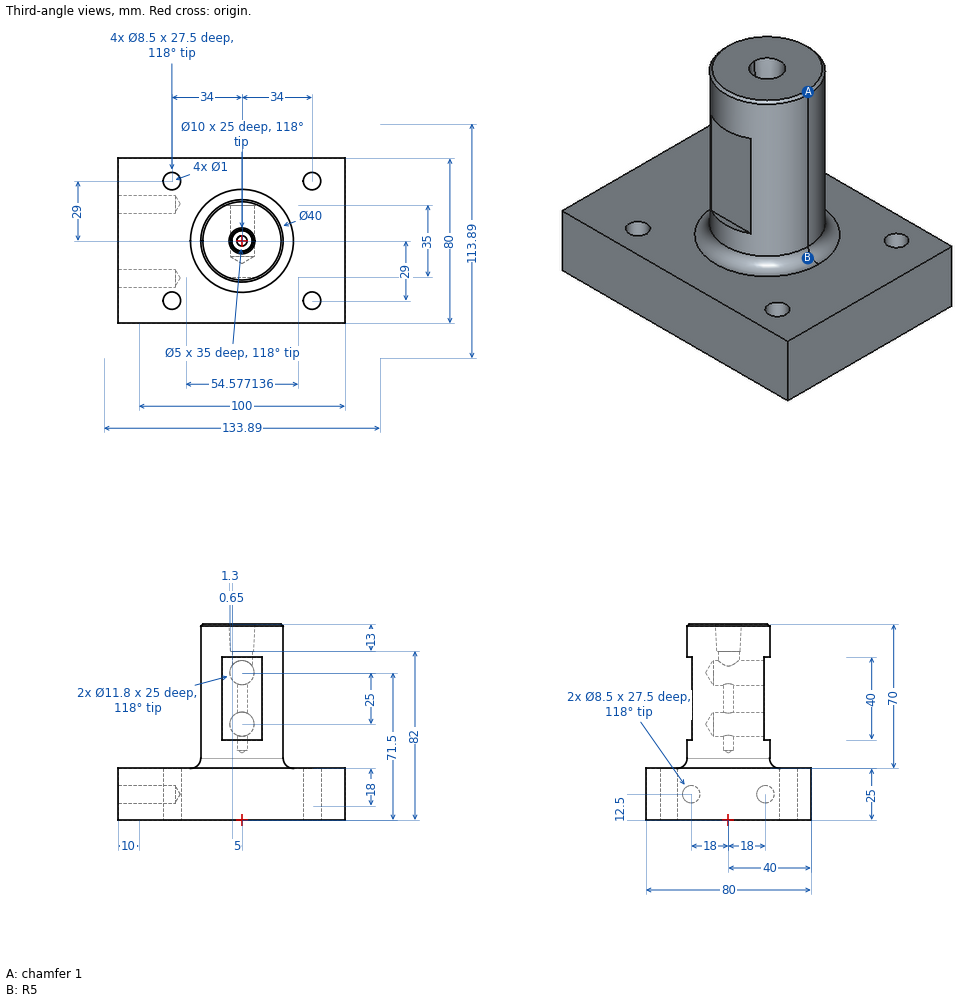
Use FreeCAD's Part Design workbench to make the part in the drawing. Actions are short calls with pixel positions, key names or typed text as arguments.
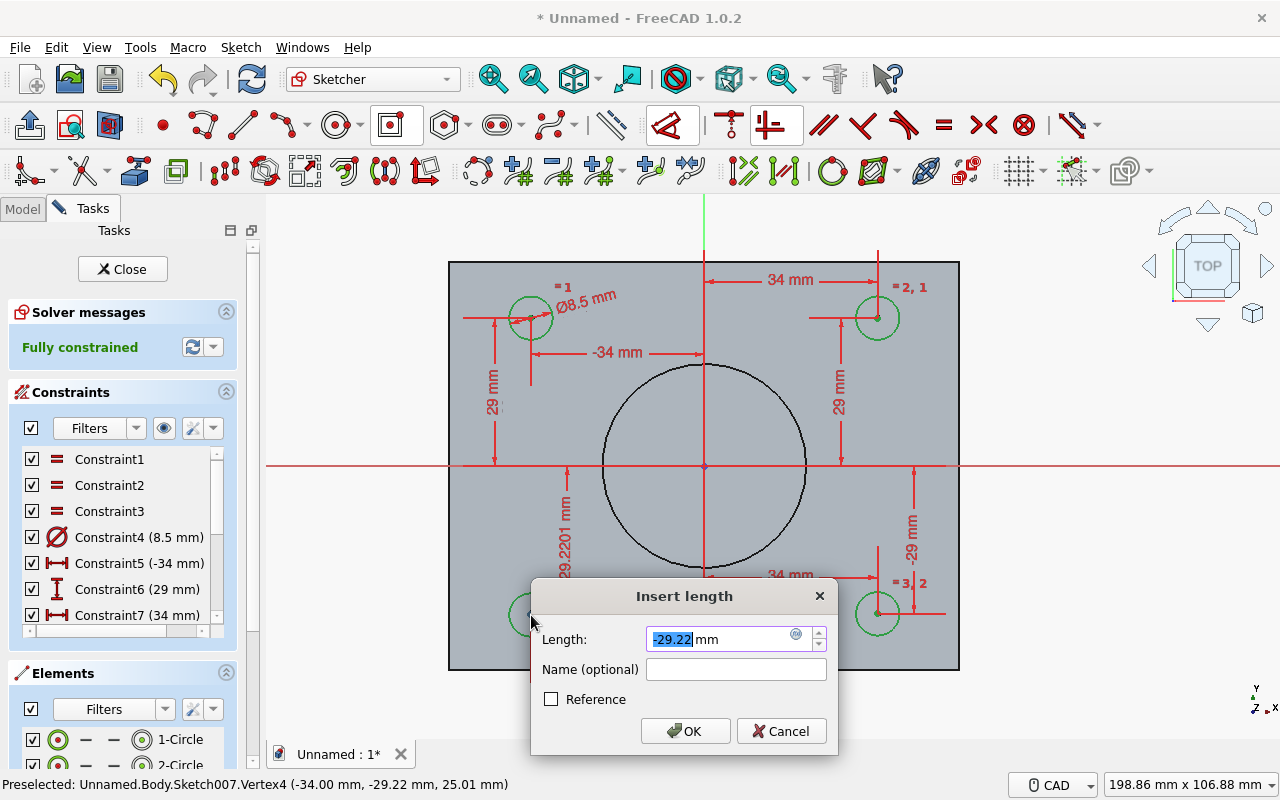
text(-29)
key(Return)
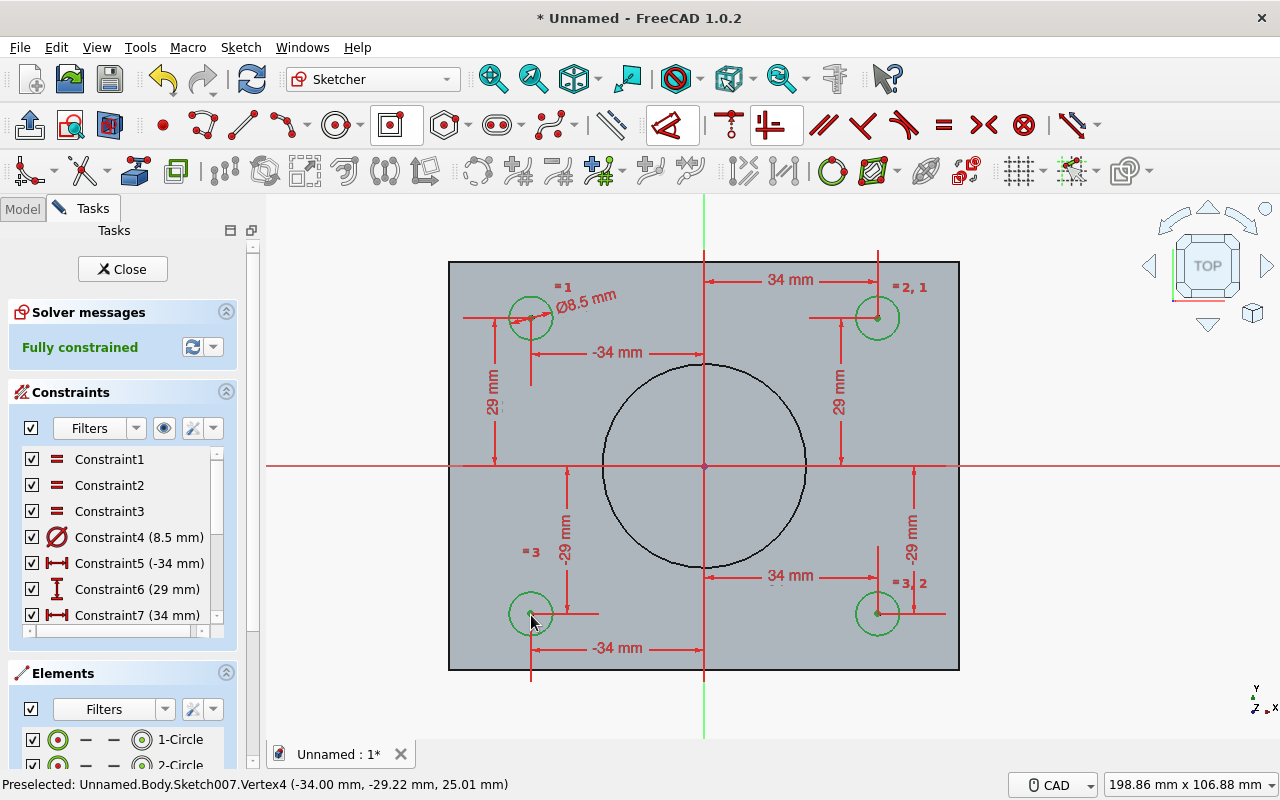
click(123, 269)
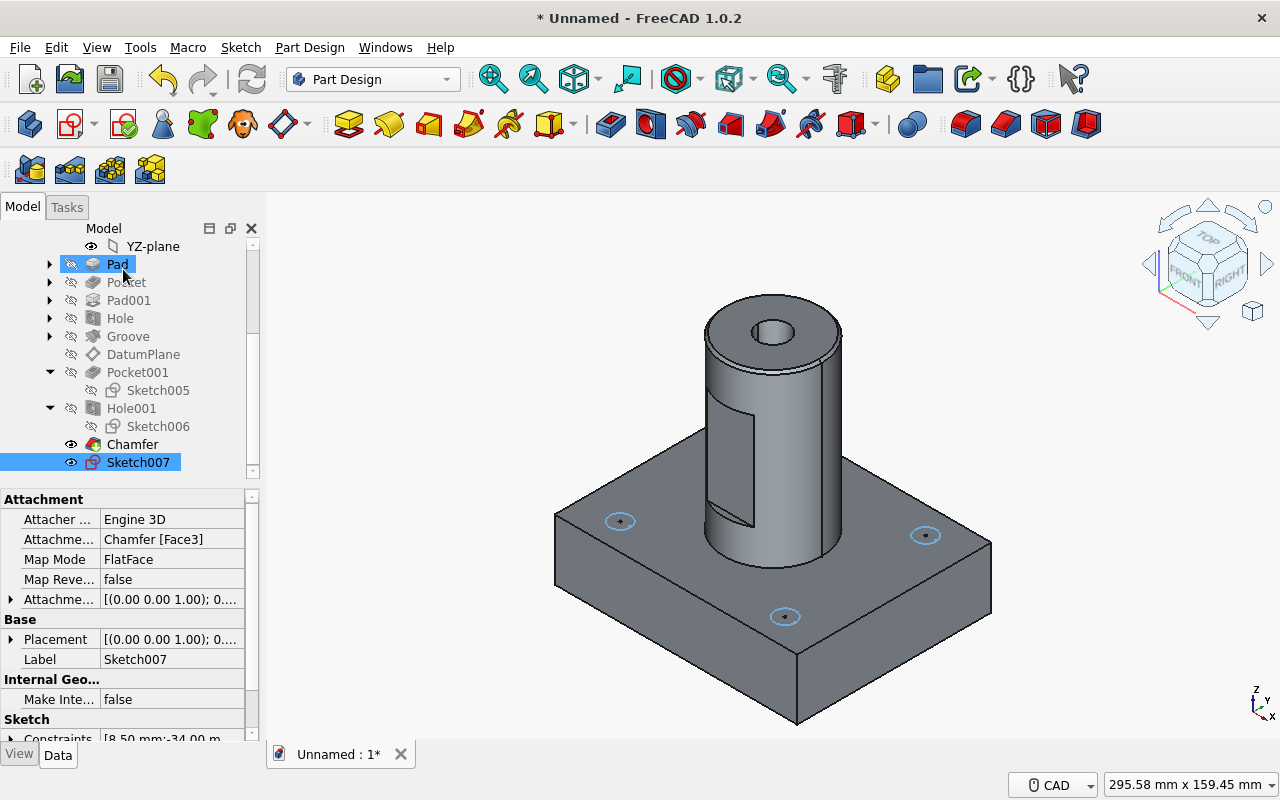
click(652, 124)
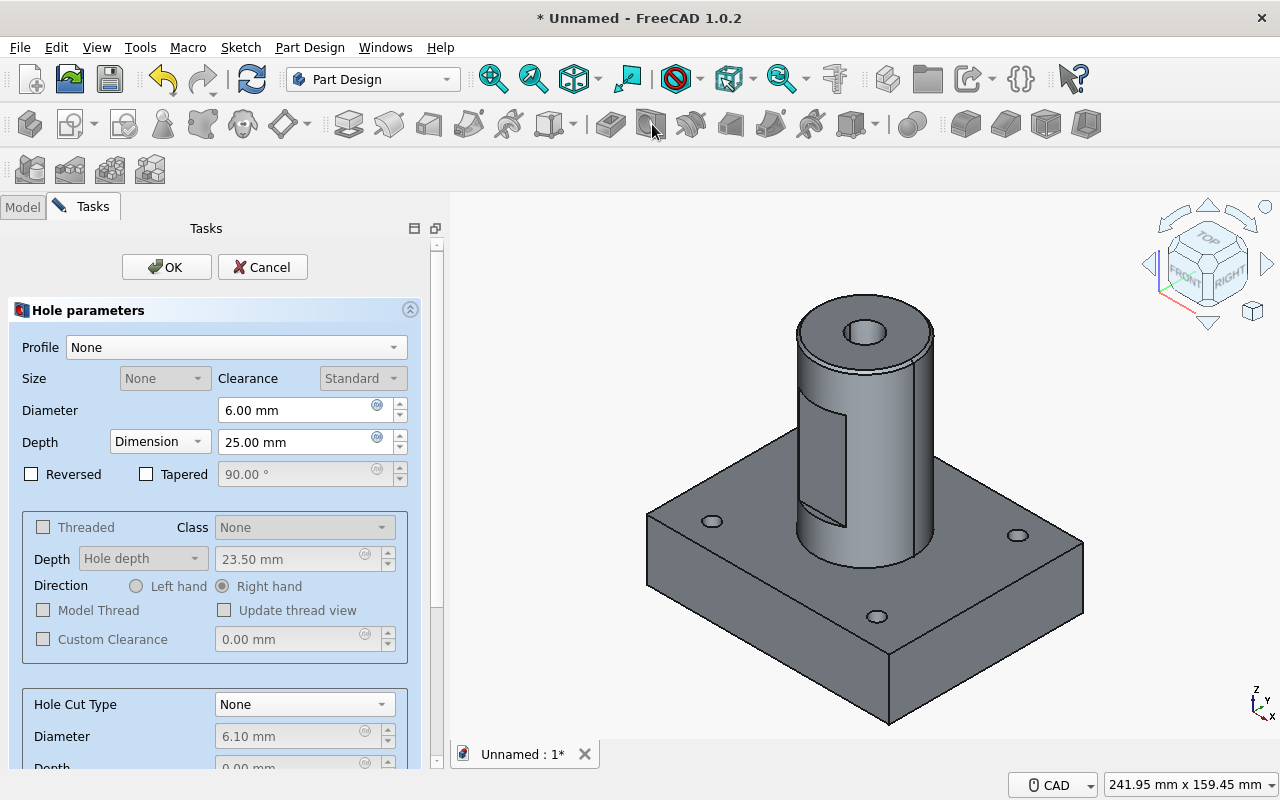
triple_click(305, 410)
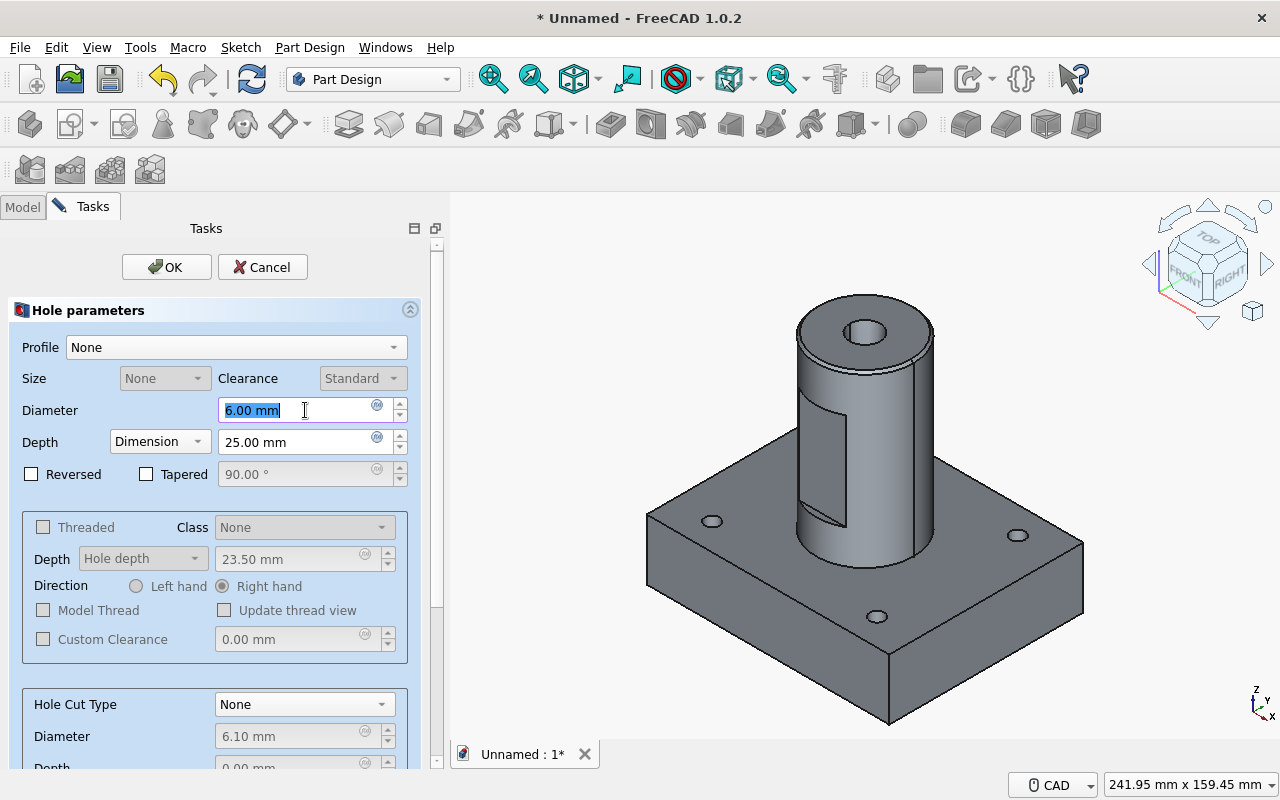
text(8.5)
key(Tab)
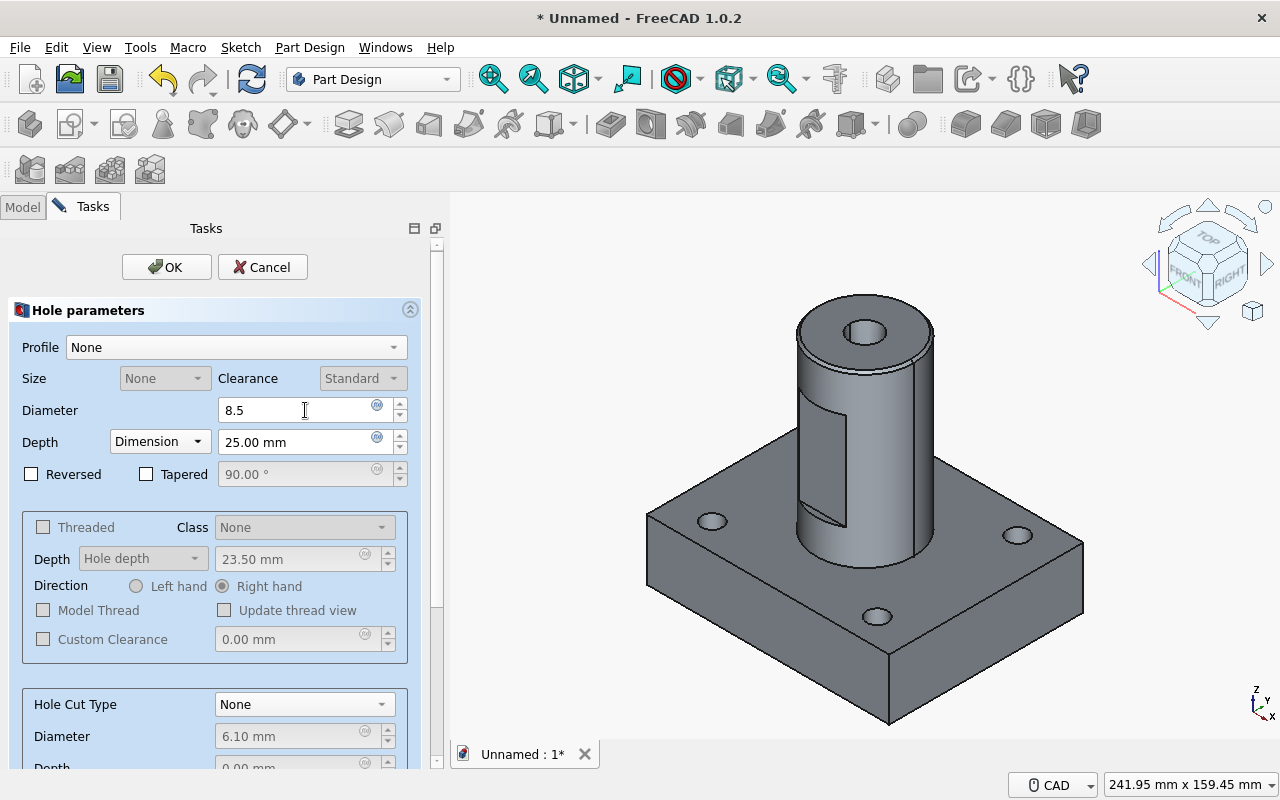
triple_click(305, 442)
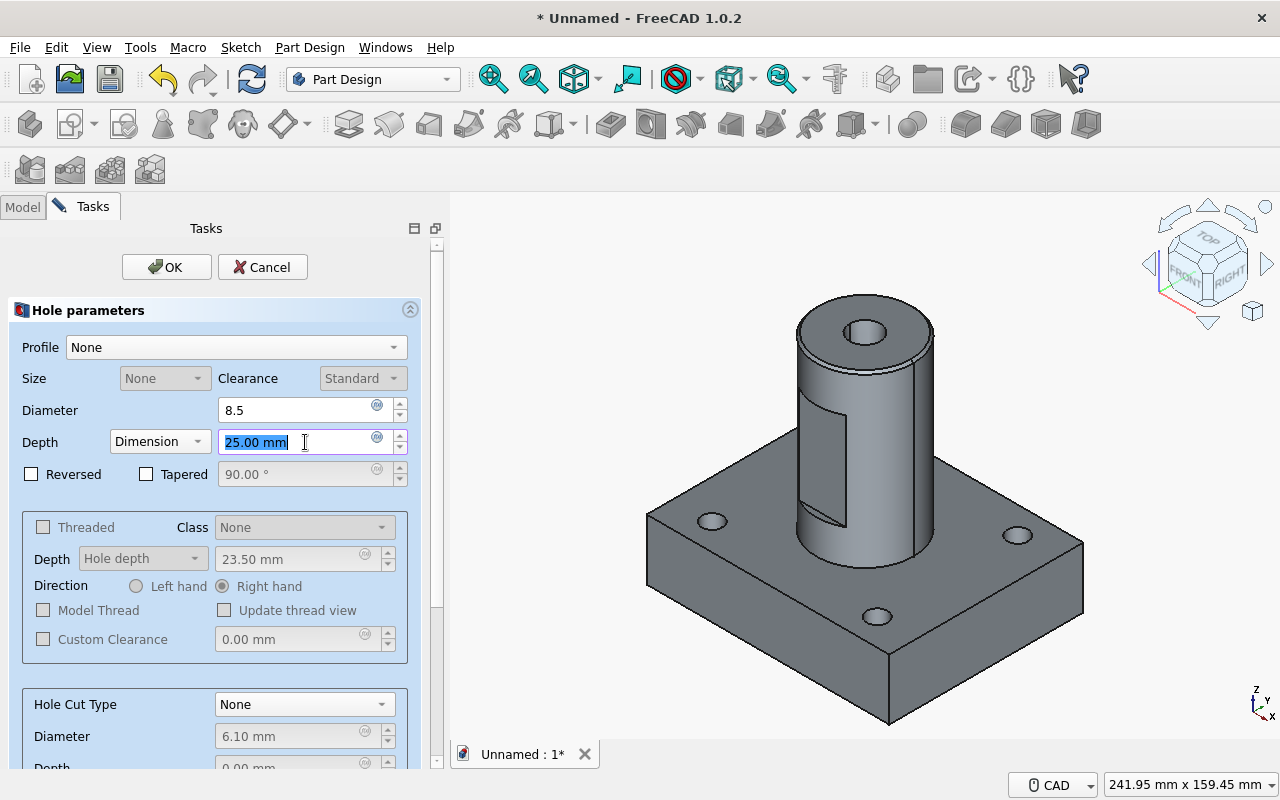
text(27.5)
key(Tab)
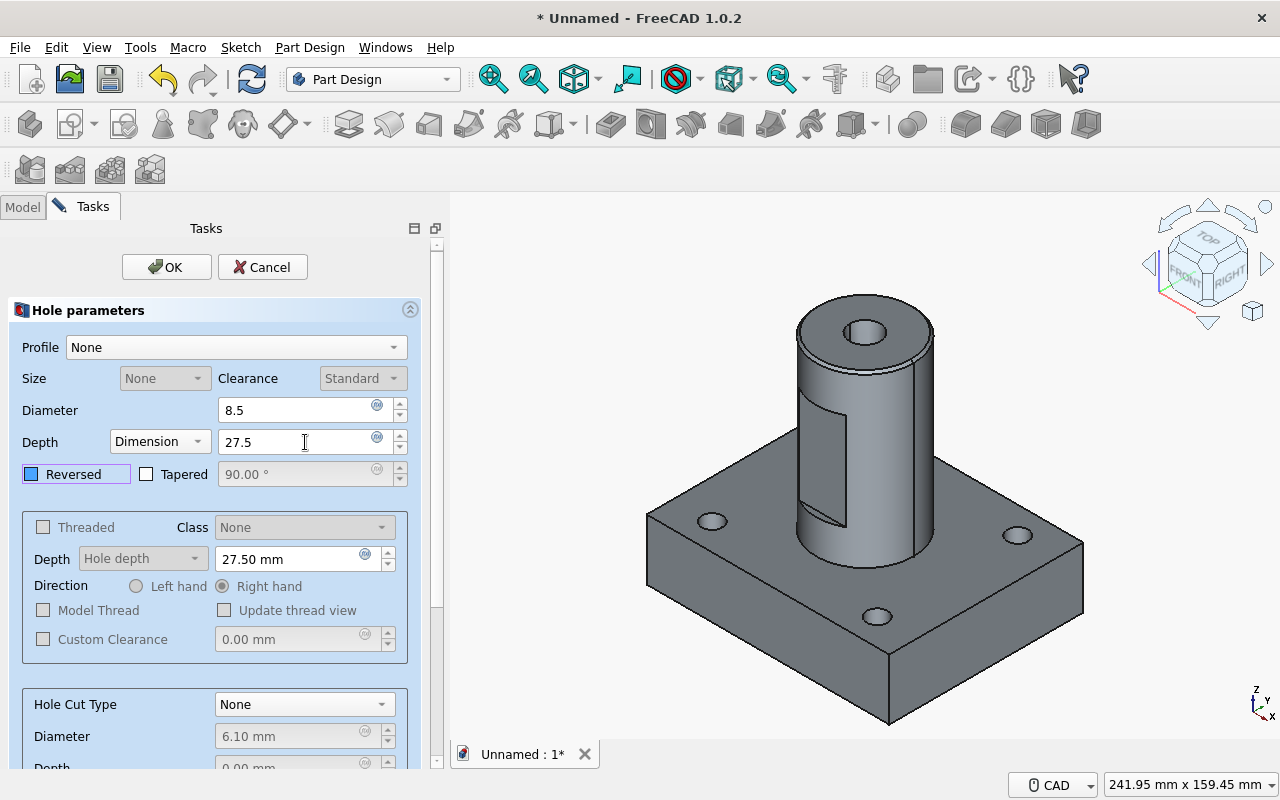
click(167, 267)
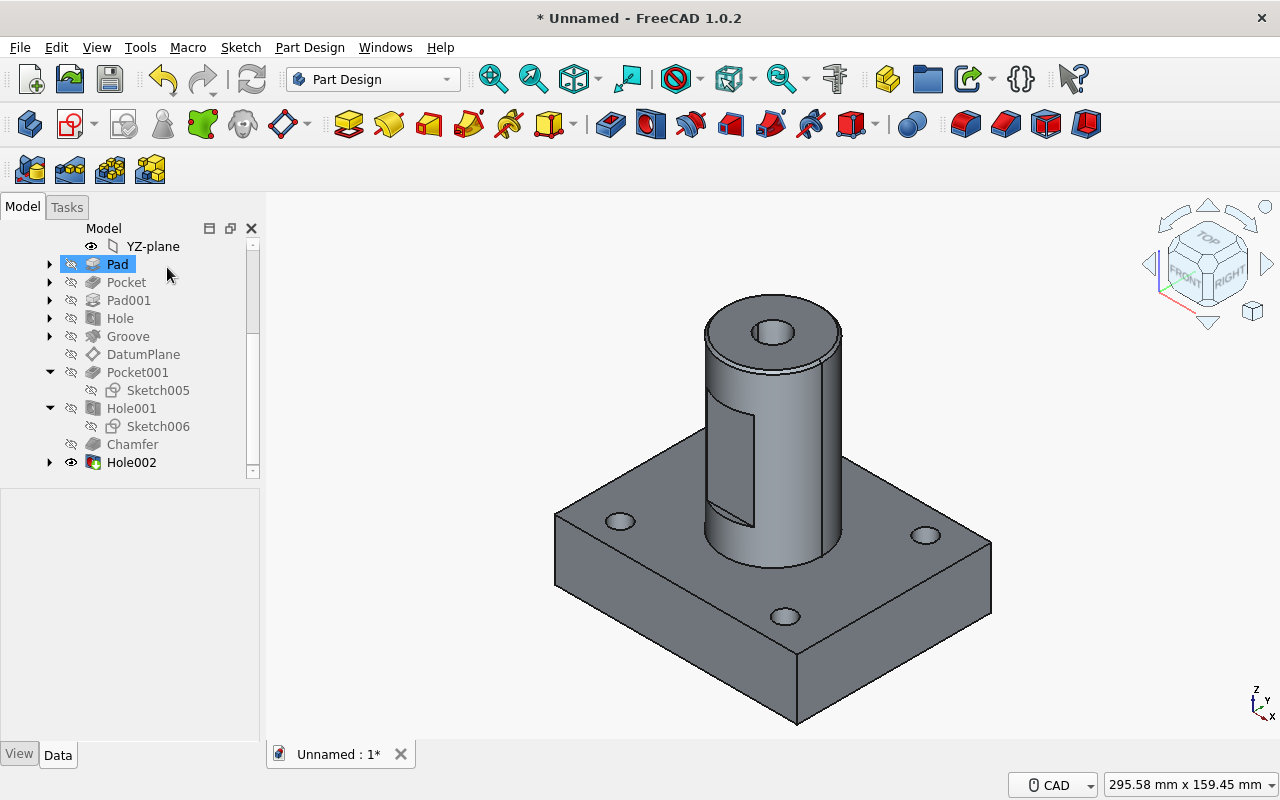
key(2)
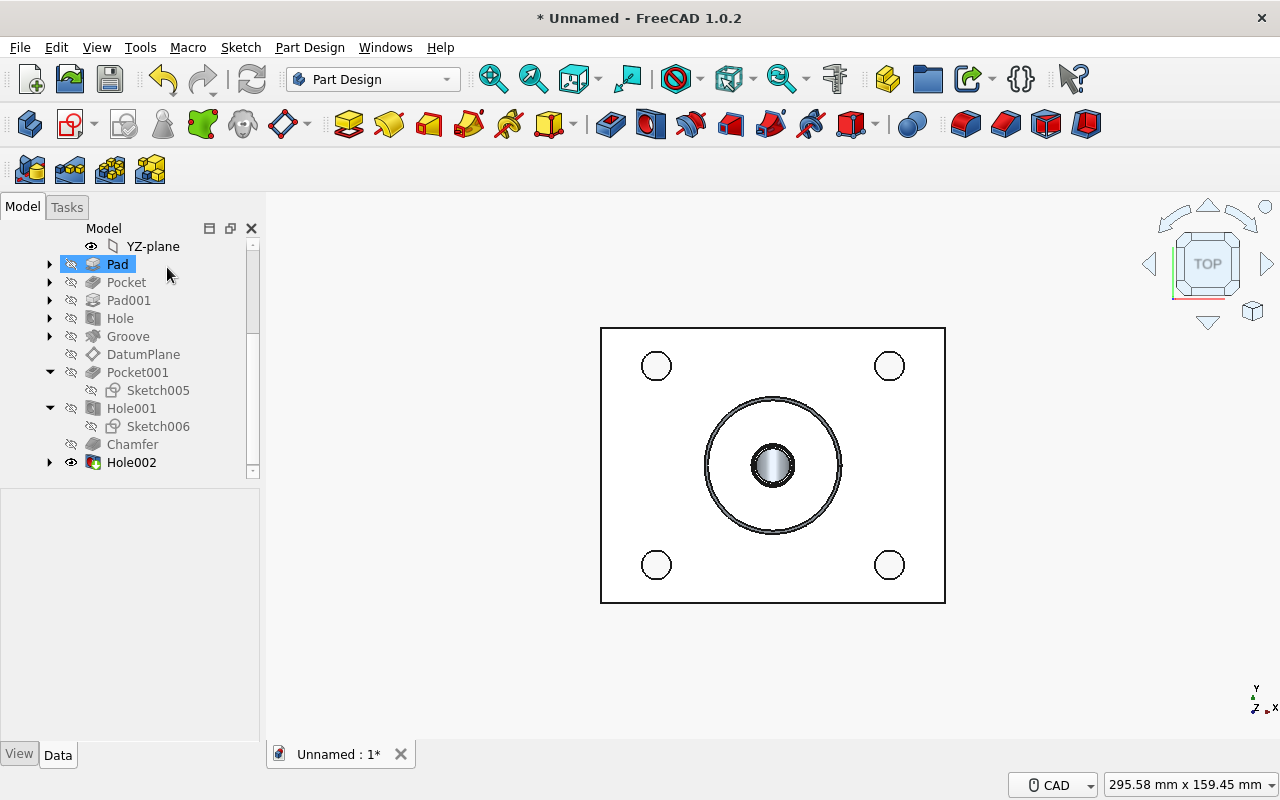
key(0)